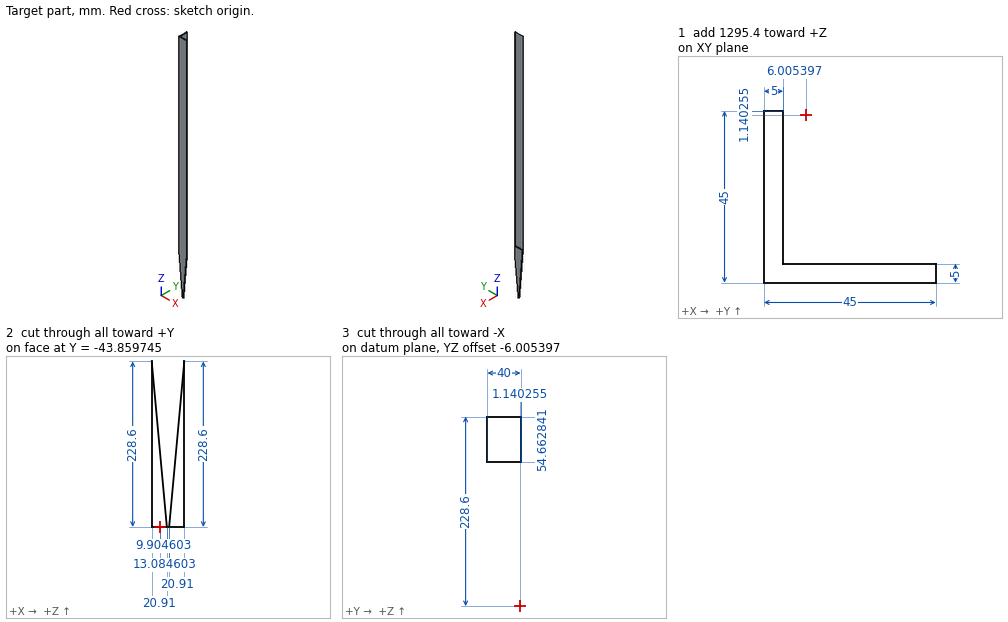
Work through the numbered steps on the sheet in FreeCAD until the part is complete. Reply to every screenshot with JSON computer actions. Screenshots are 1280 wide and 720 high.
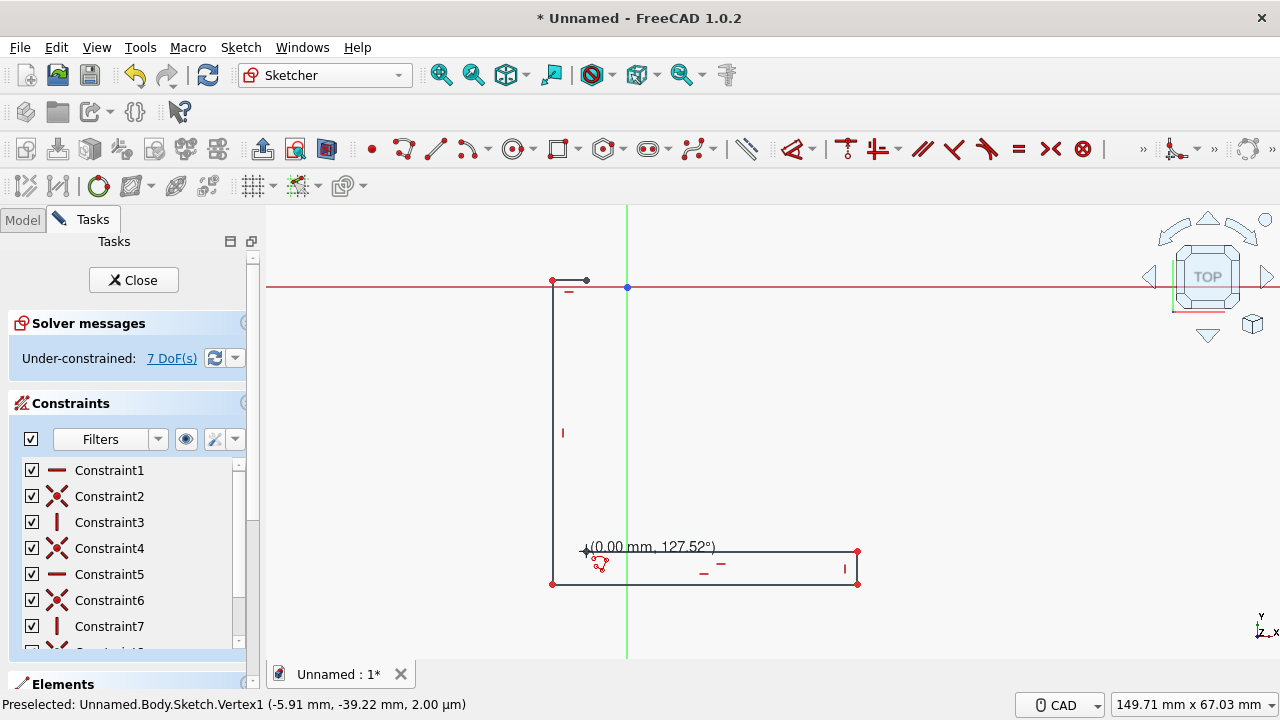
{"action": "scroll", "coordinate": [586, 280], "scroll_direction": "up", "scroll_amount": 4}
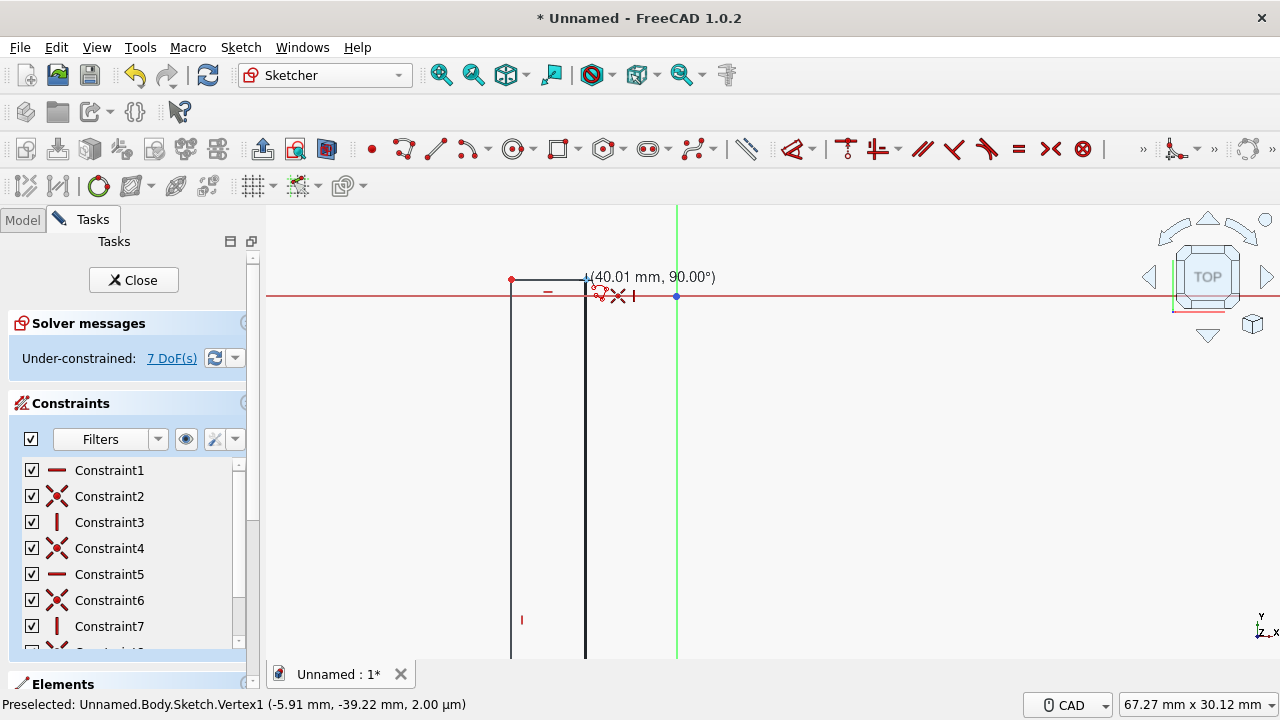
{"action": "left_click", "coordinate": [586, 280]}
{"action": "key", "text": "Escape"}
{"action": "key", "text": "Escape"}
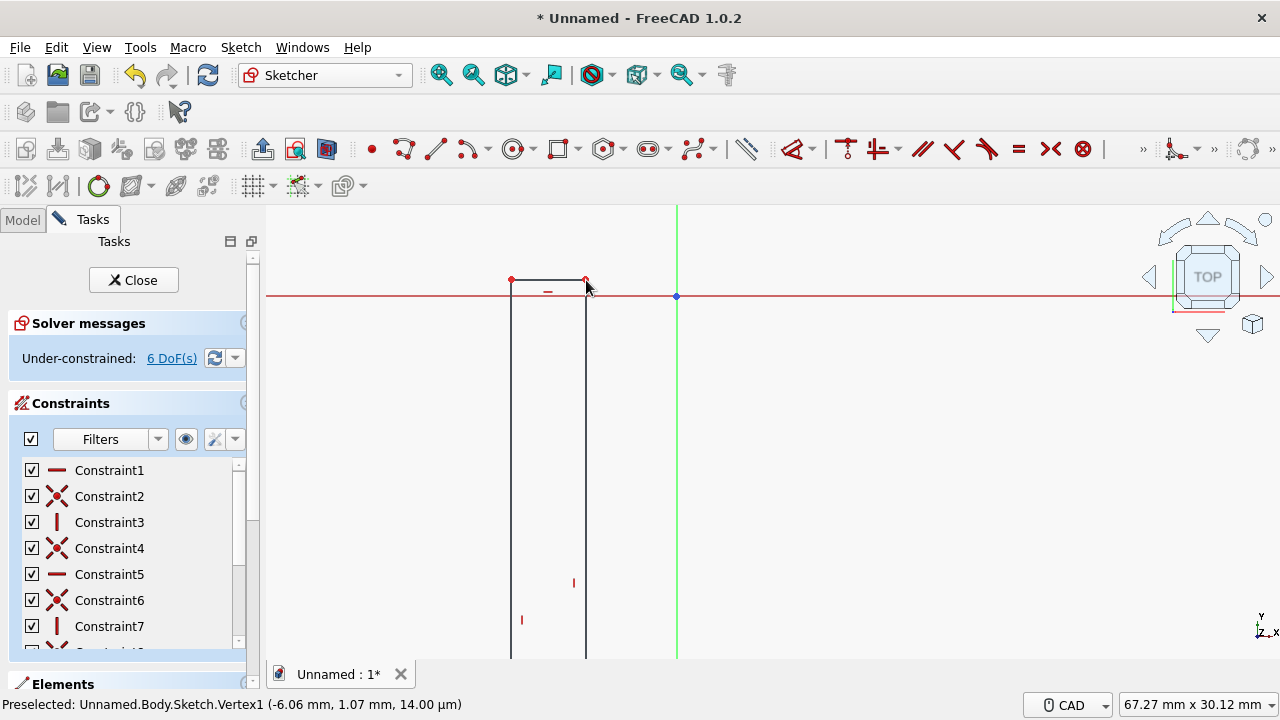
{"action": "left_click", "coordinate": [792, 150]}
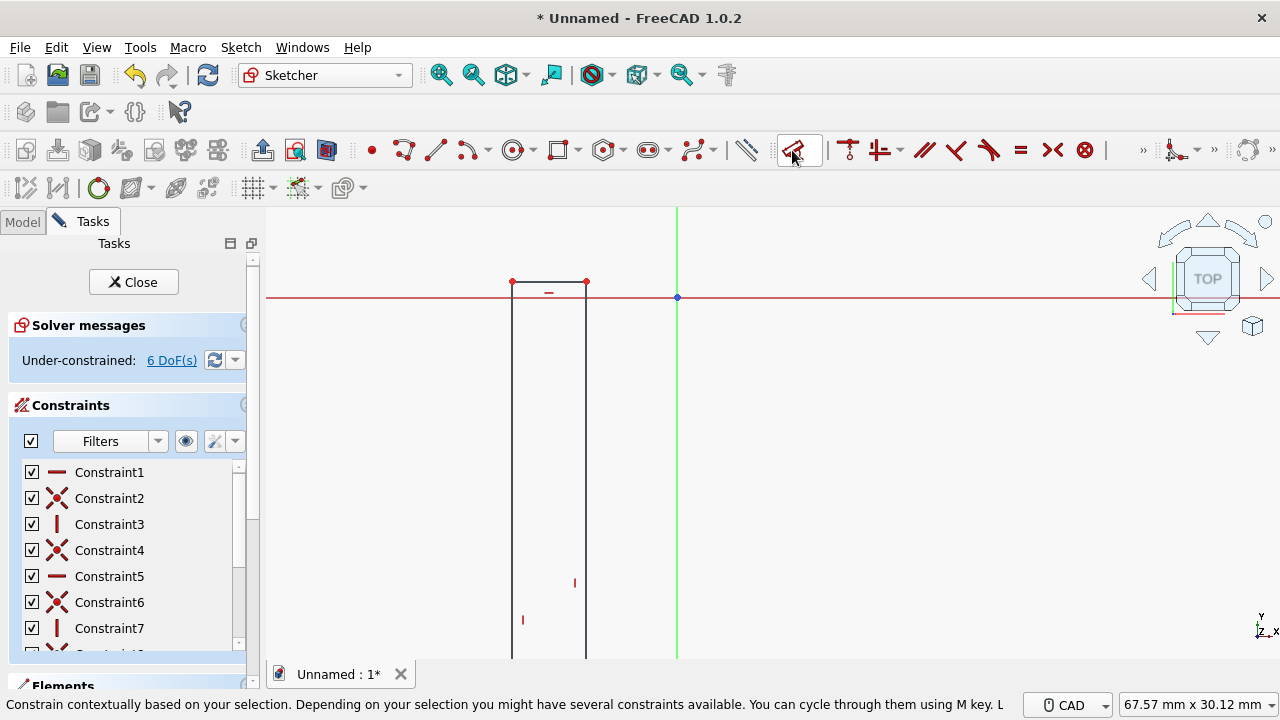
{"action": "left_click", "coordinate": [564, 282]}
{"action": "left_click", "coordinate": [549, 248]}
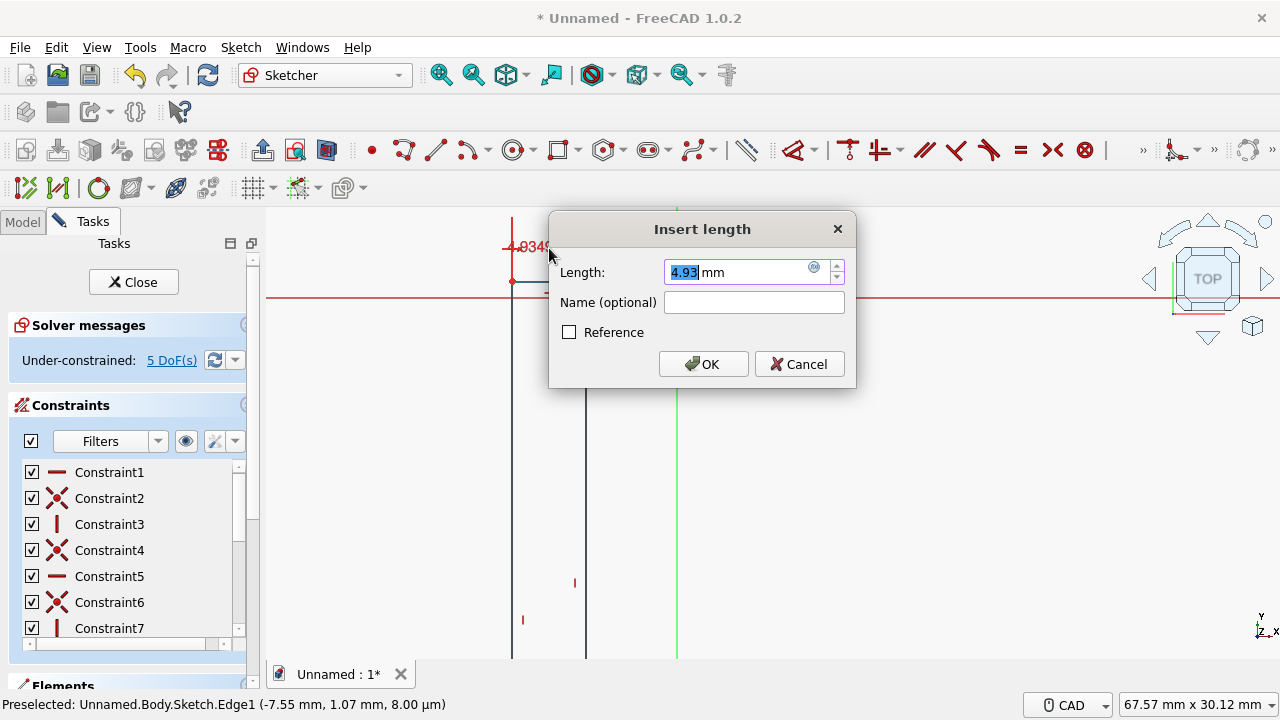
{"action": "type", "text": "5"}
{"action": "key", "text": "Return"}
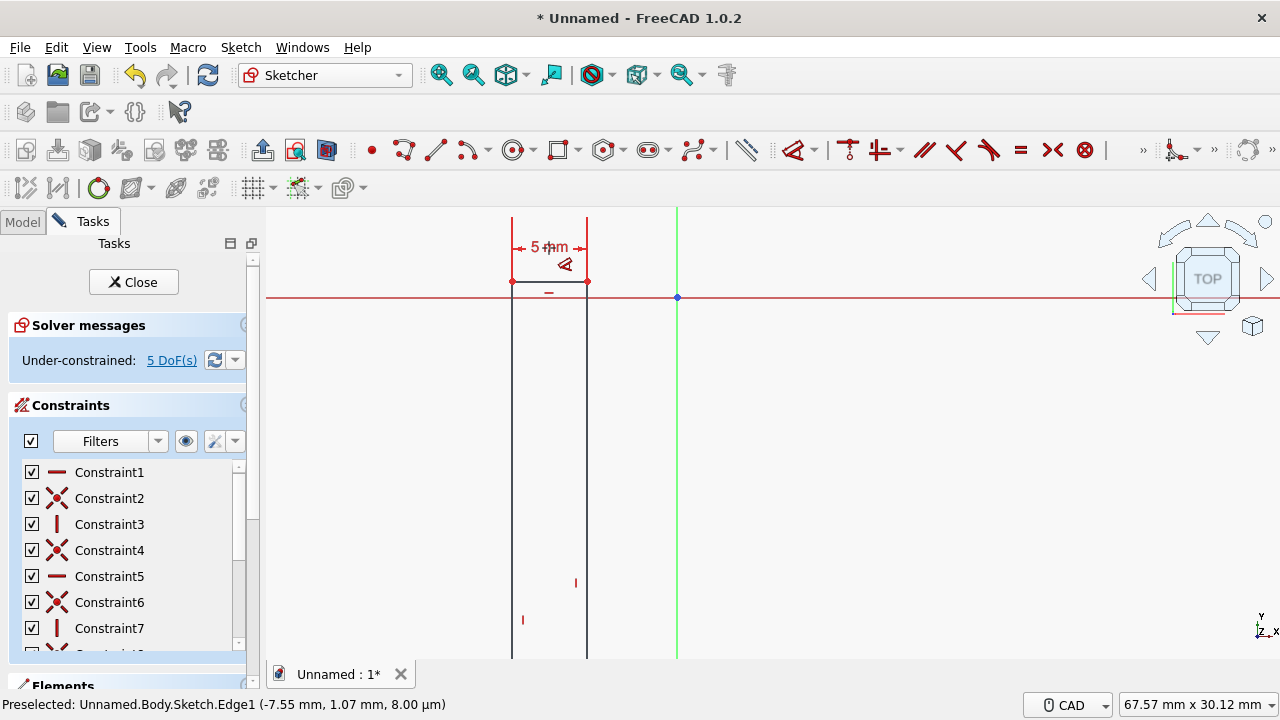
{"action": "scroll", "coordinate": [586, 282], "scroll_direction": "down", "scroll_amount": 4}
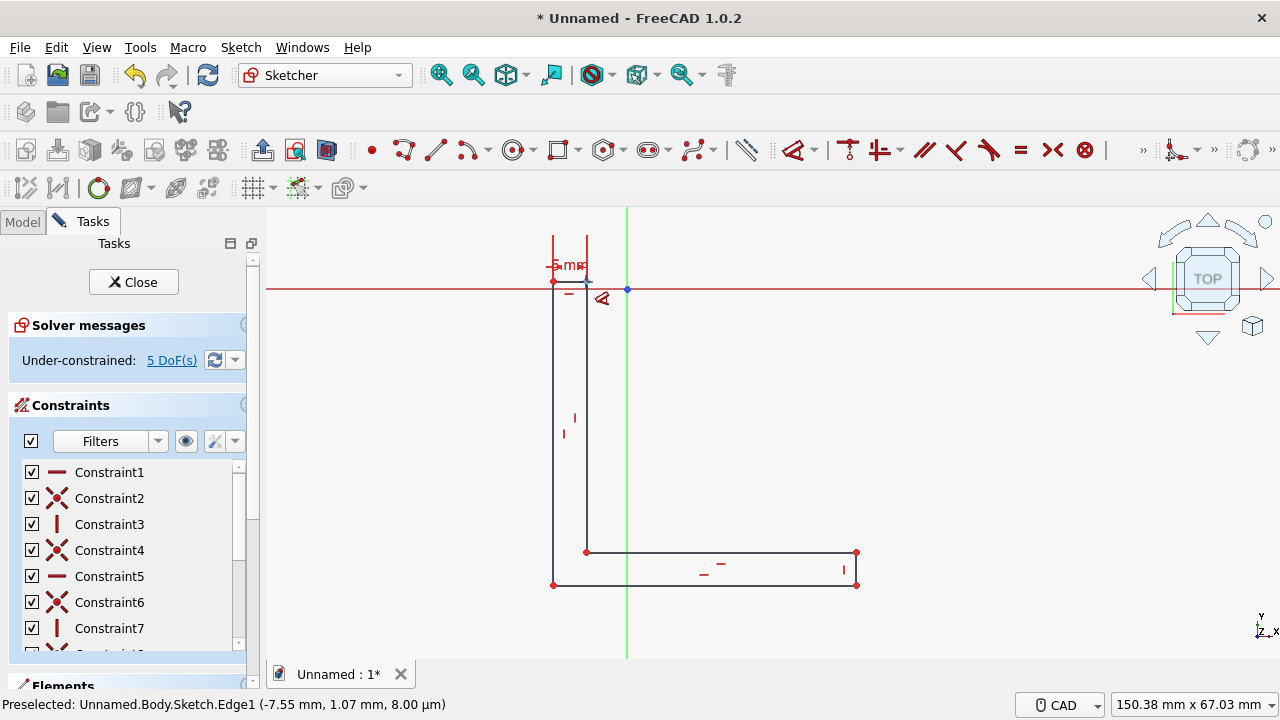
{"action": "scroll", "coordinate": [856, 576], "scroll_direction": "up", "scroll_amount": 2}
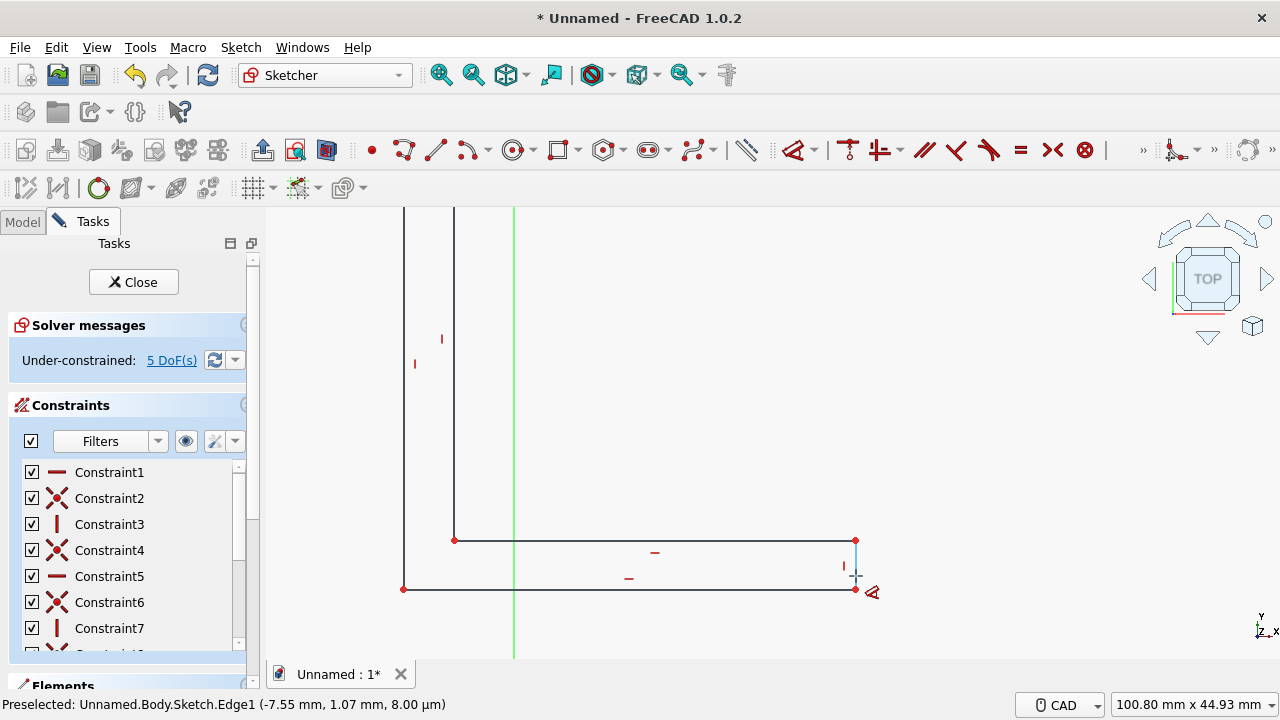
{"action": "left_click", "coordinate": [856, 575]}
{"action": "left_click", "coordinate": [890, 565]}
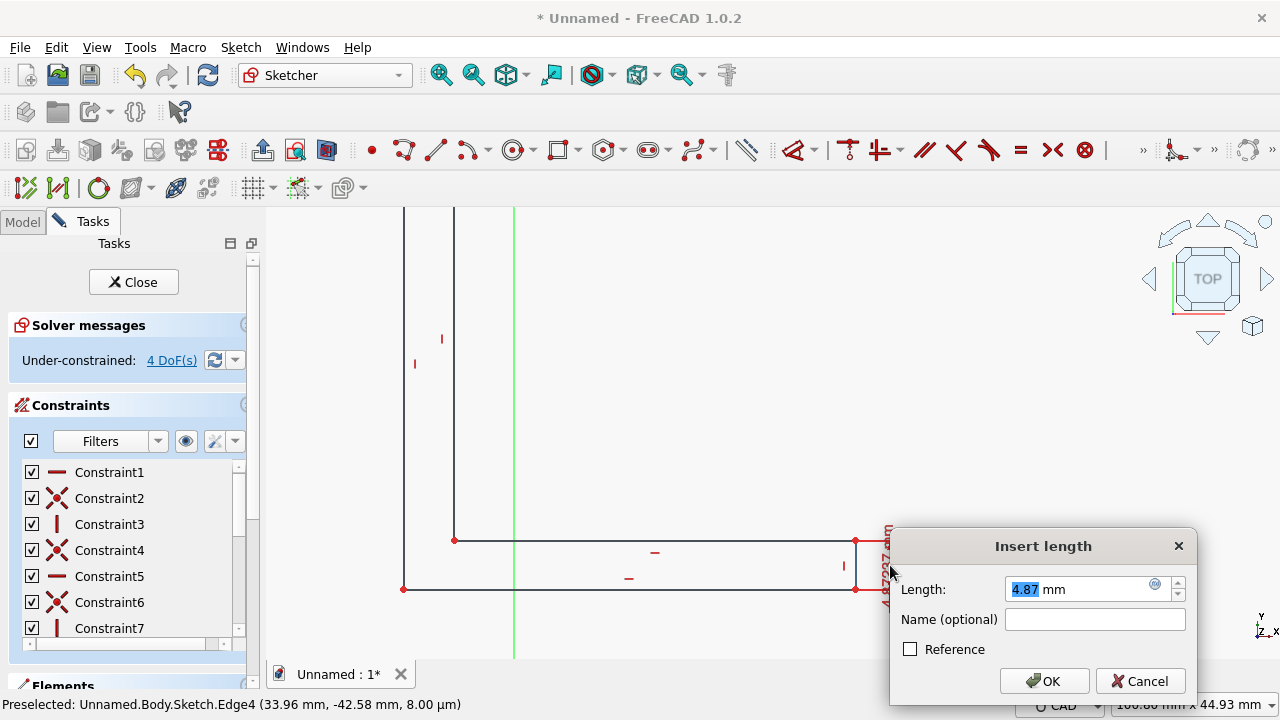
{"action": "type", "text": "5"}
{"action": "key", "text": "Return"}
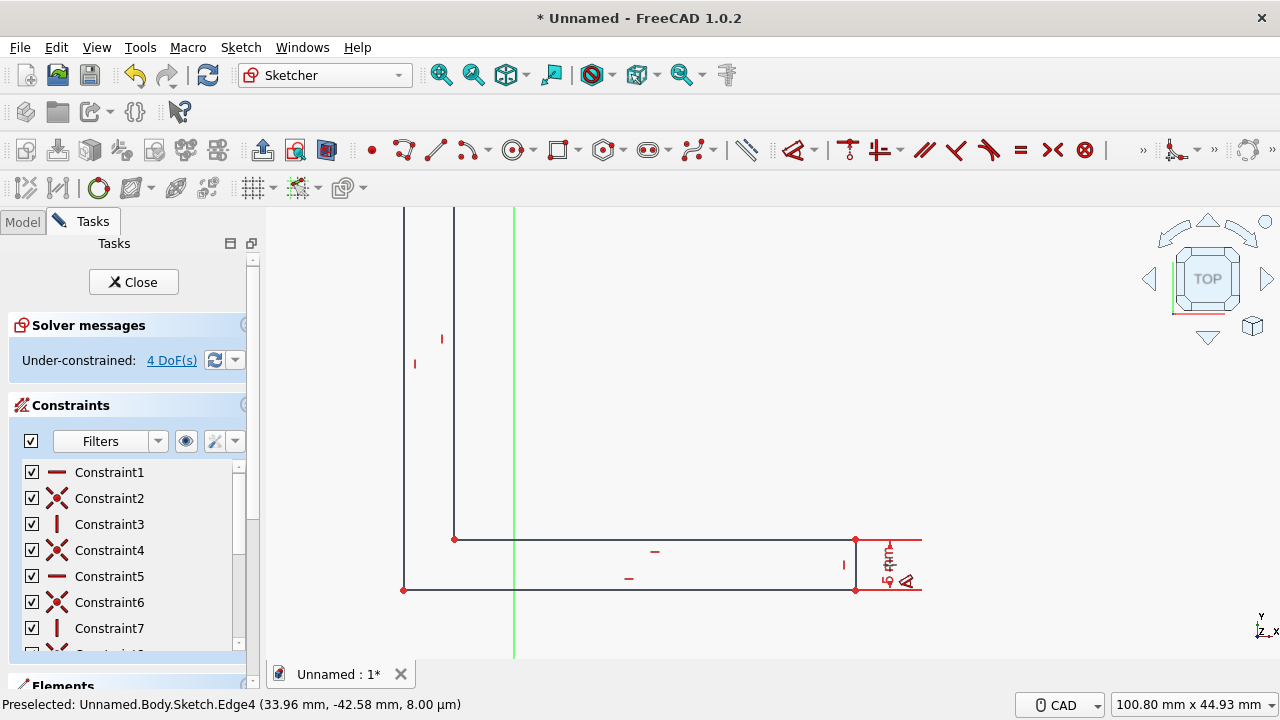
{"action": "left_click", "coordinate": [404, 273]}
{"action": "left_click", "coordinate": [370, 413]}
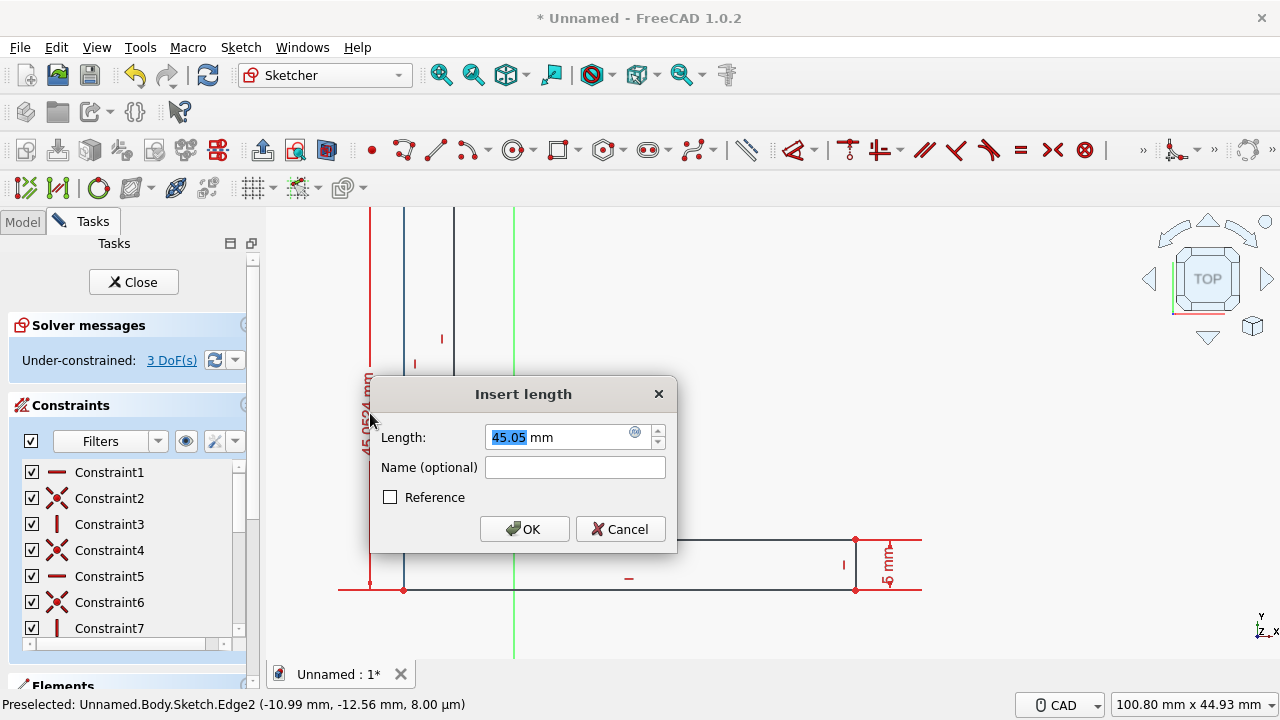
{"action": "type", "text": "45"}
{"action": "key", "text": "Return"}